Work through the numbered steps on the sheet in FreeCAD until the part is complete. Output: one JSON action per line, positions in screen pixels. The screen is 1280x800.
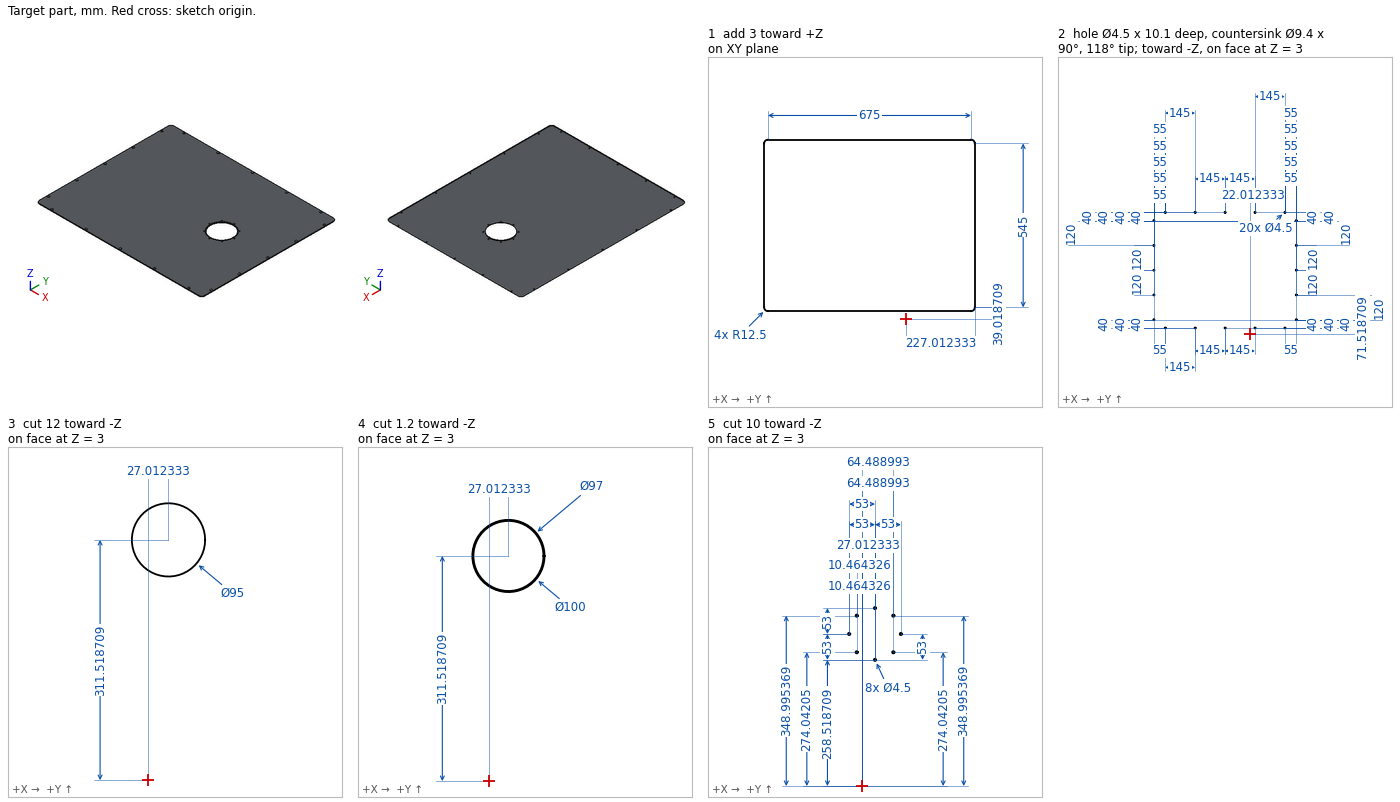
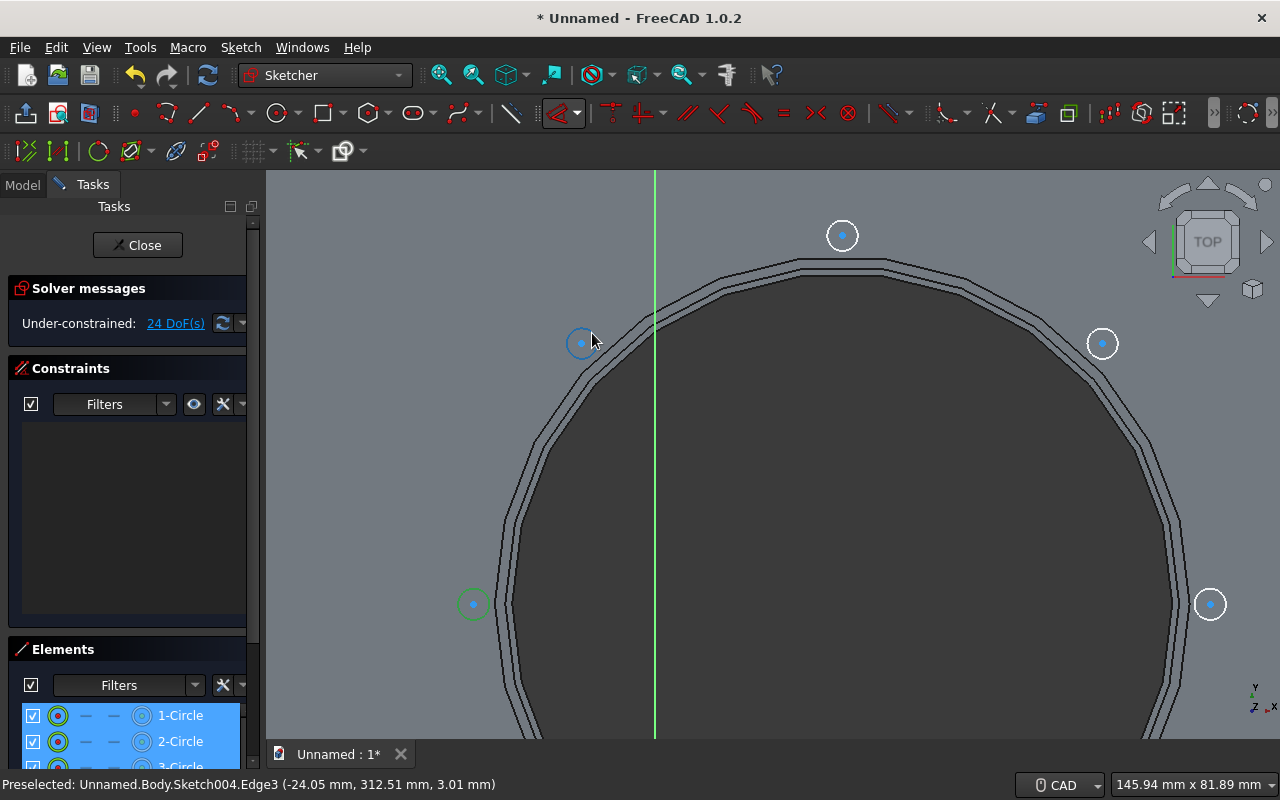
{"action": "left_click", "coordinate": [593, 333]}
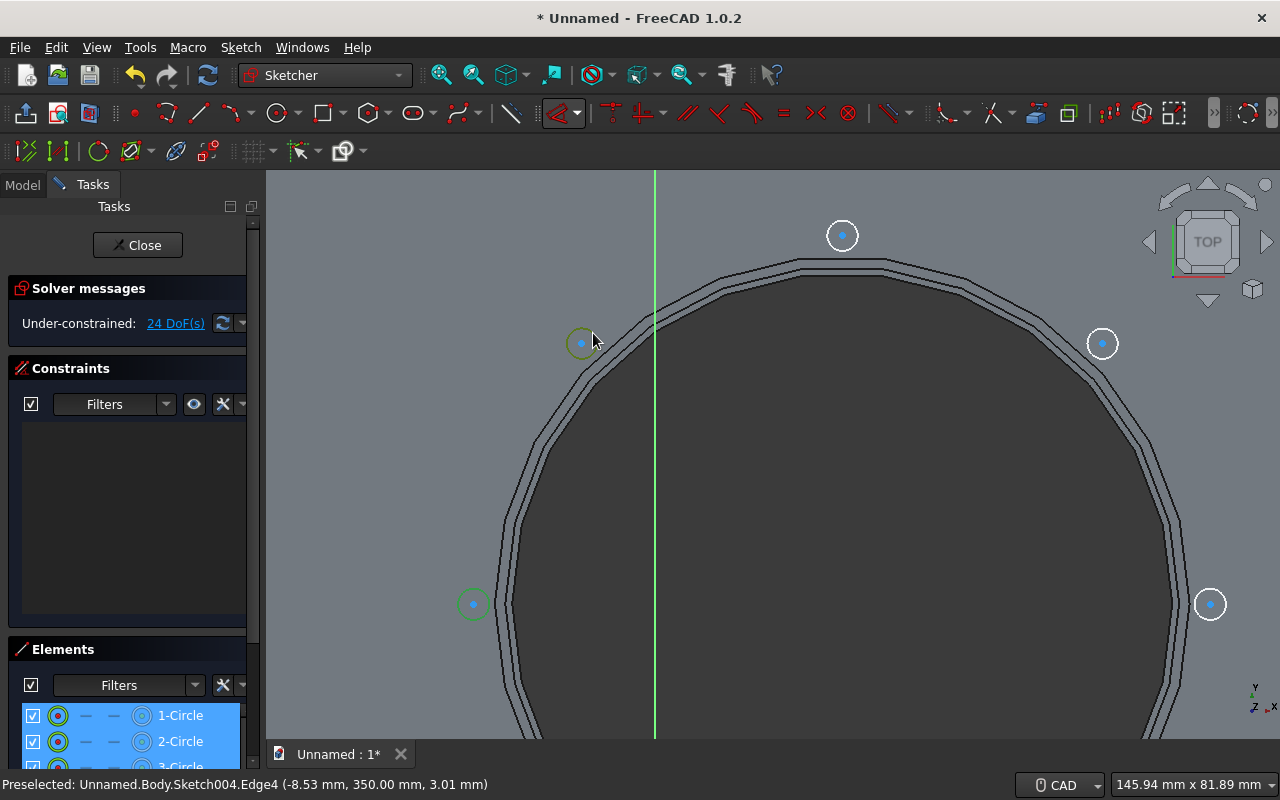
{"action": "left_click", "coordinate": [853, 225]}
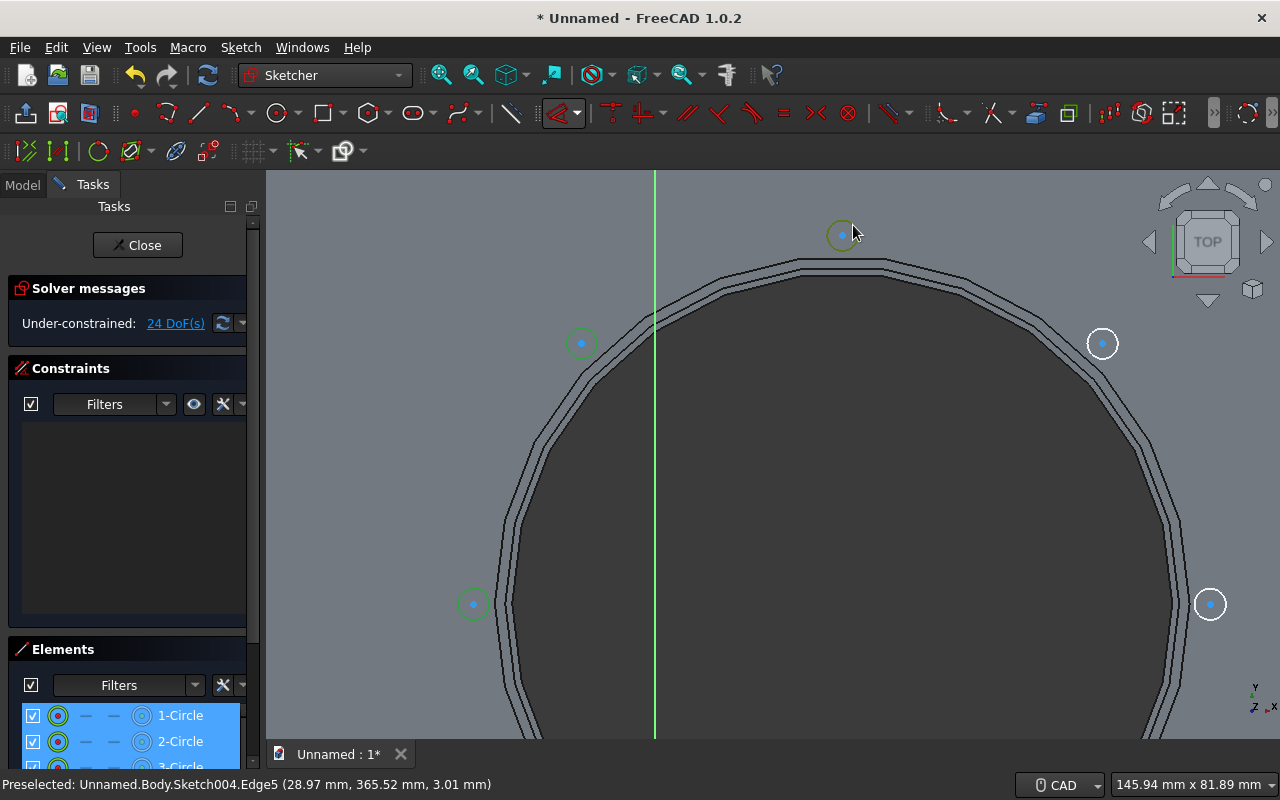
{"action": "left_click", "coordinate": [1113, 333]}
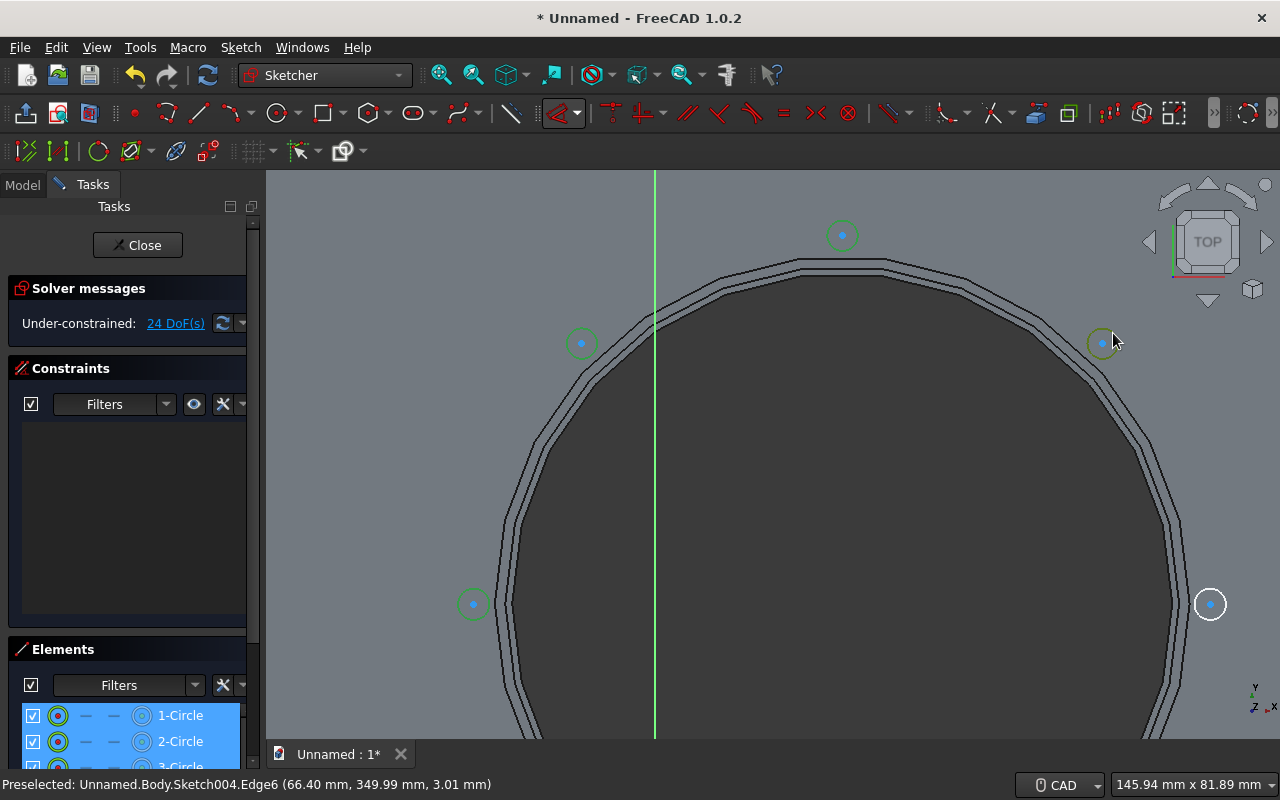
{"action": "scroll", "coordinate": [592, 333], "scroll_direction": "down", "scroll_amount": 4}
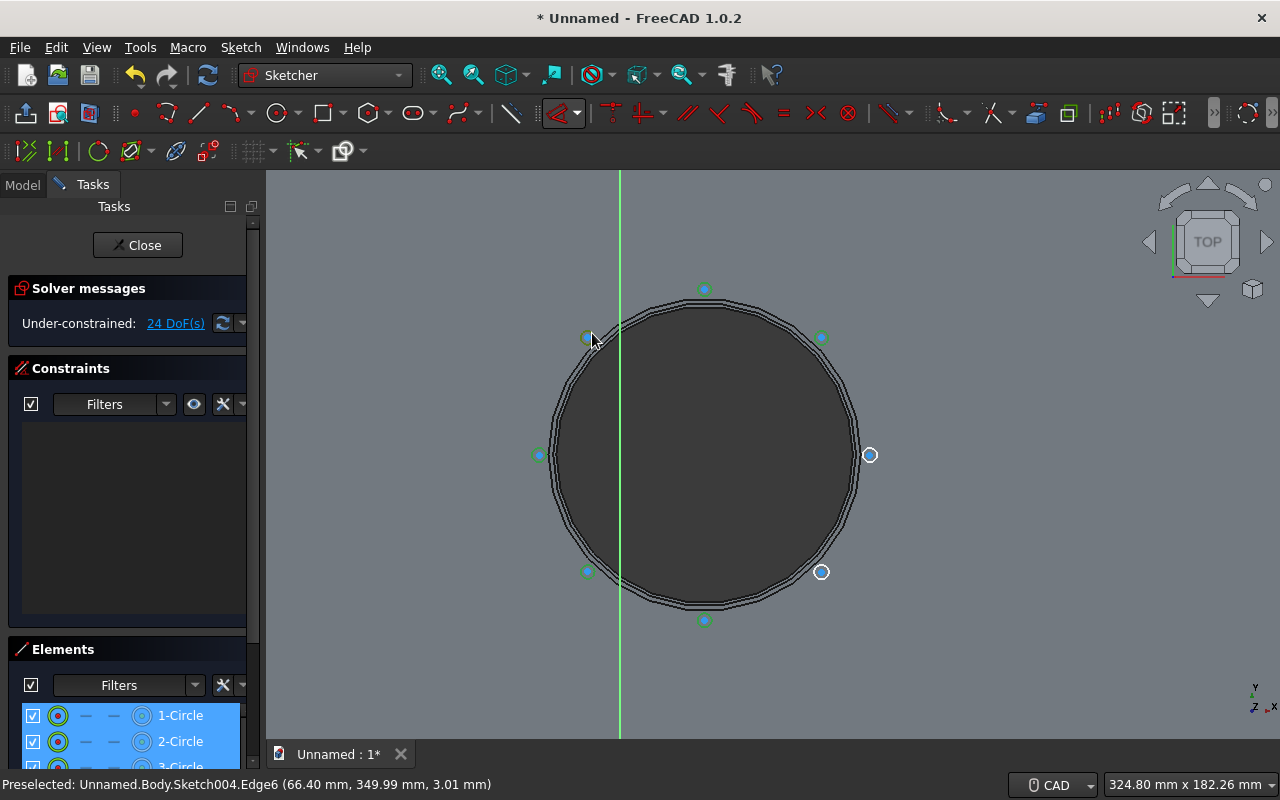
{"action": "scroll", "coordinate": [875, 450], "scroll_direction": "up", "scroll_amount": 4}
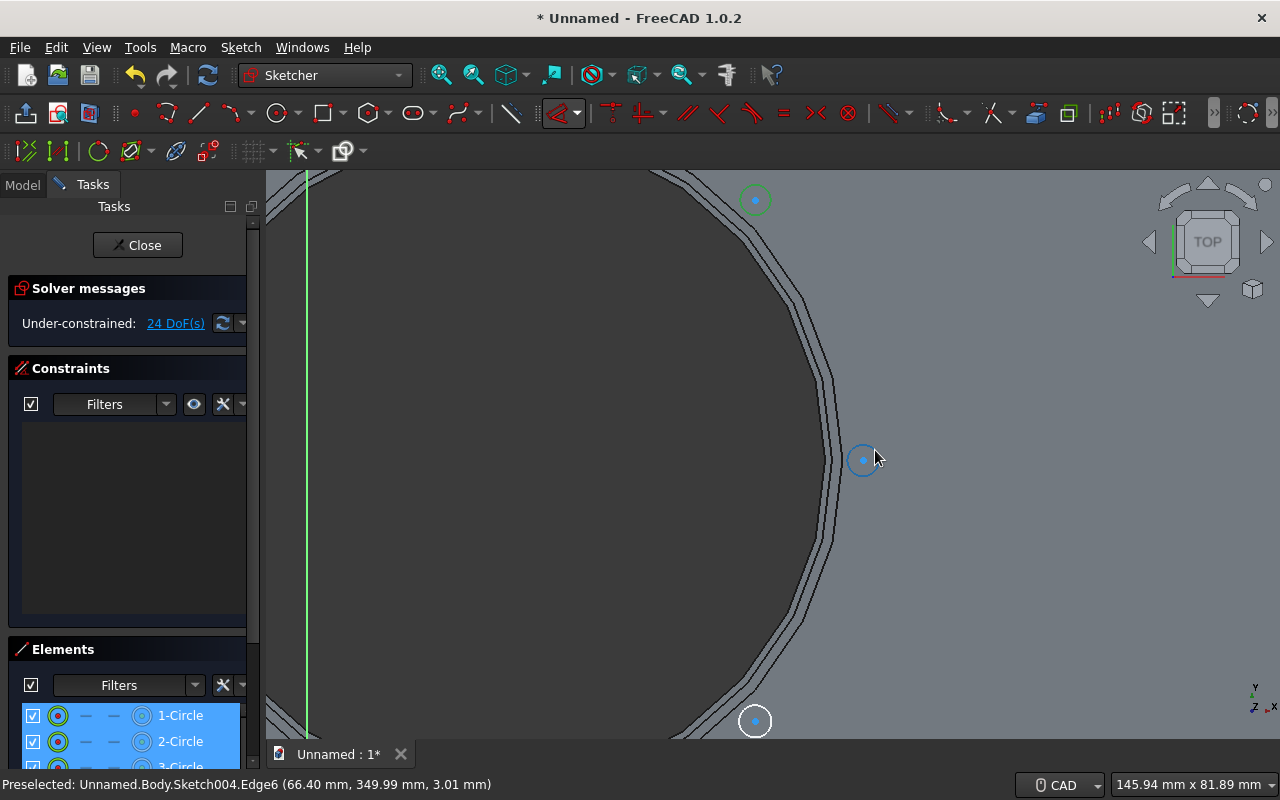
{"action": "left_click", "coordinate": [874, 450]}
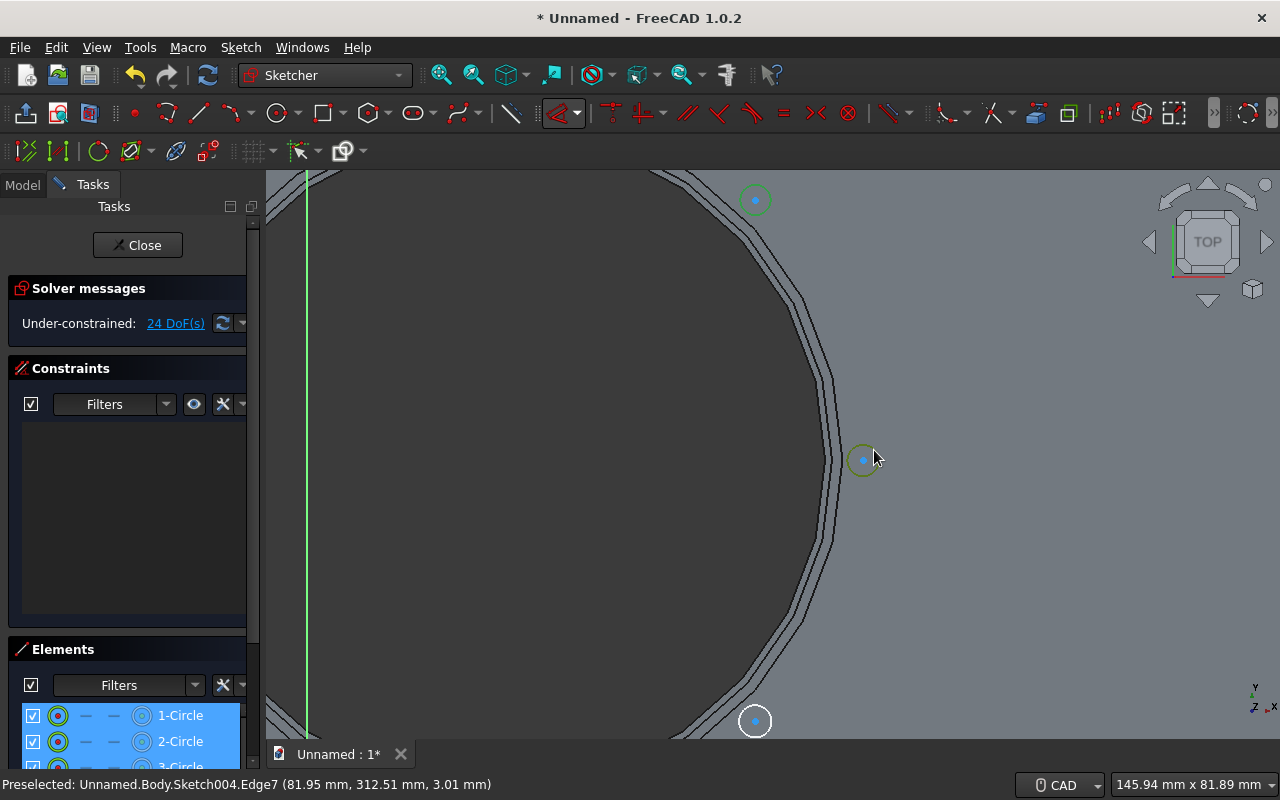
{"action": "left_click", "coordinate": [767, 710]}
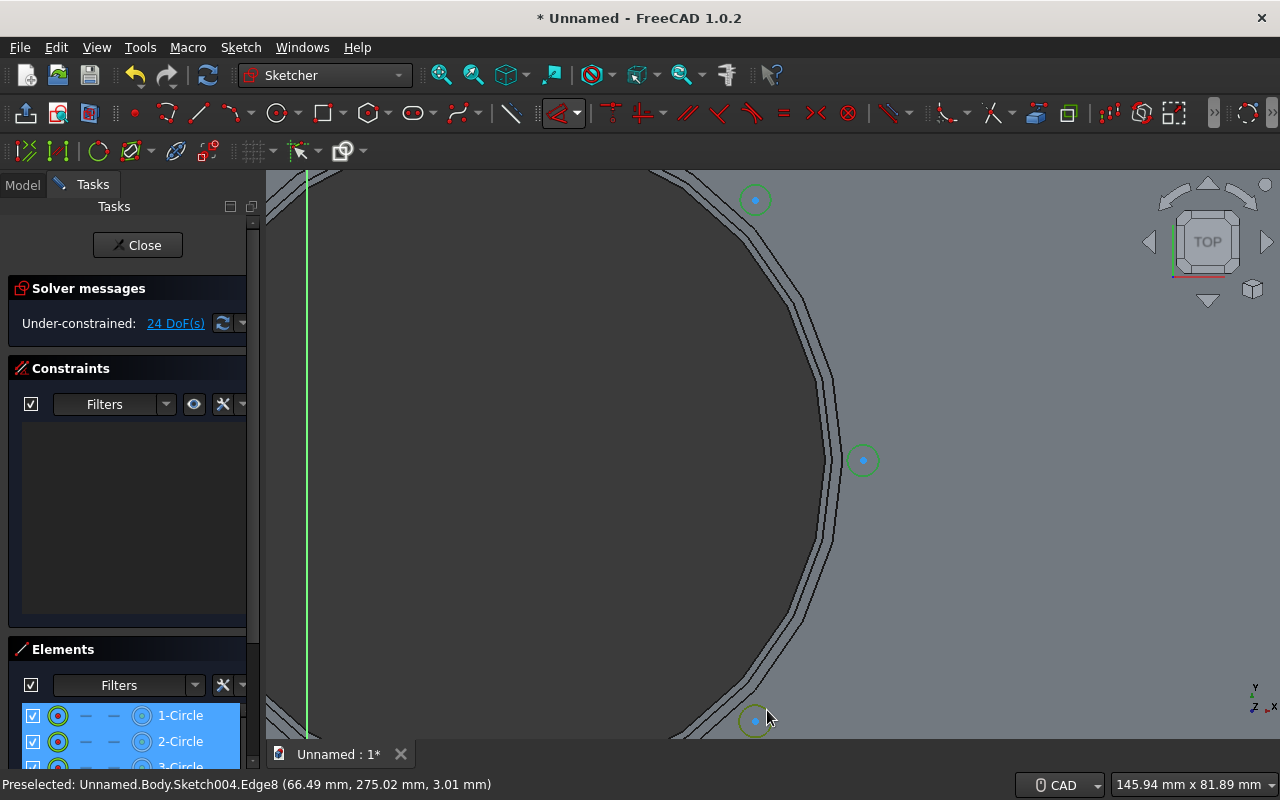
{"action": "left_click", "coordinate": [784, 114]}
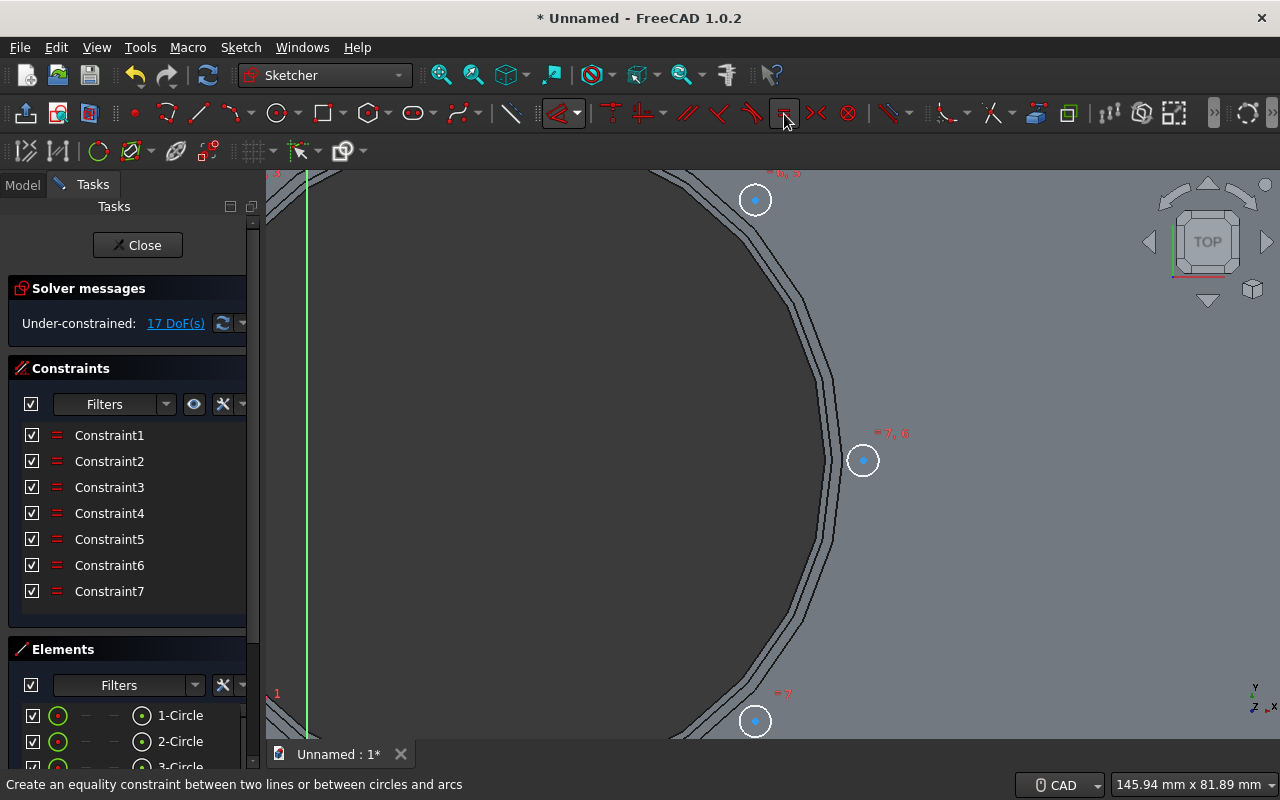
{"action": "scroll", "coordinate": [875, 450], "scroll_direction": "down", "scroll_amount": 4}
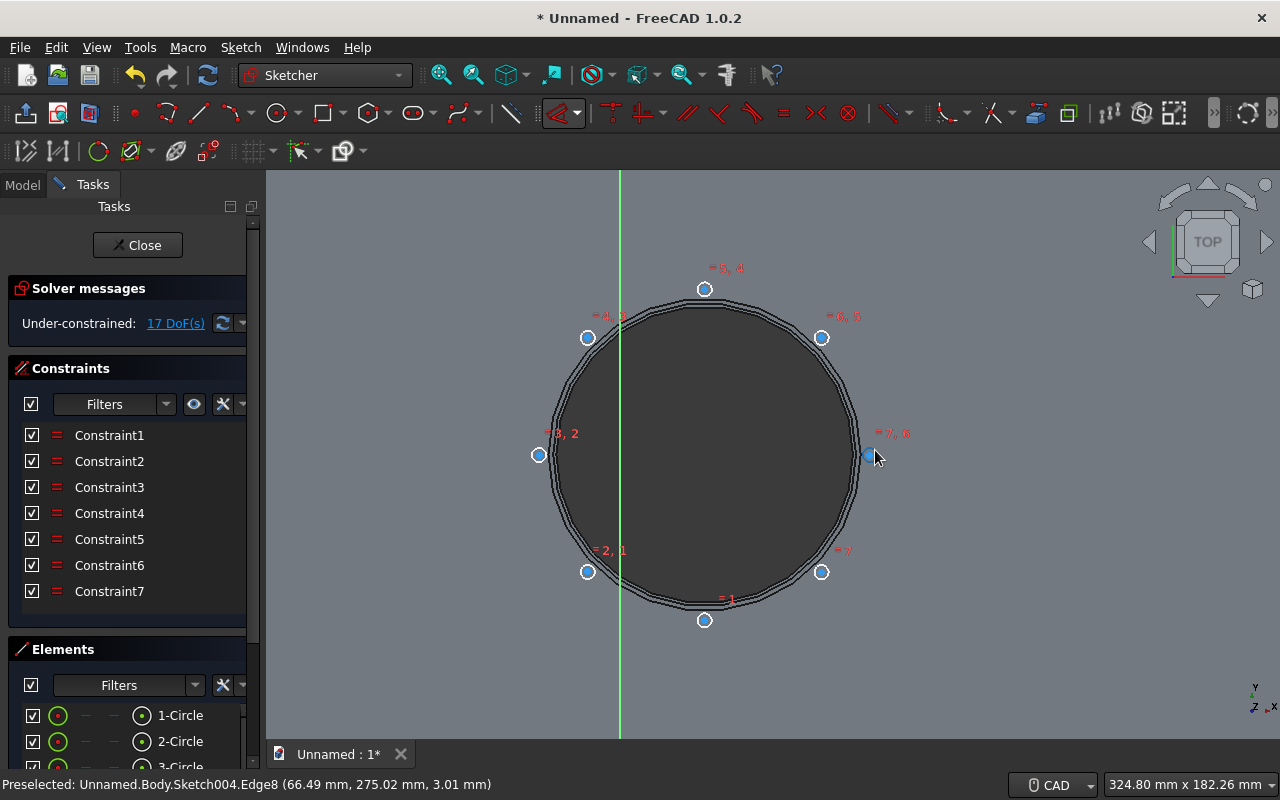
{"action": "scroll", "coordinate": [710, 615], "scroll_direction": "up", "scroll_amount": 6}